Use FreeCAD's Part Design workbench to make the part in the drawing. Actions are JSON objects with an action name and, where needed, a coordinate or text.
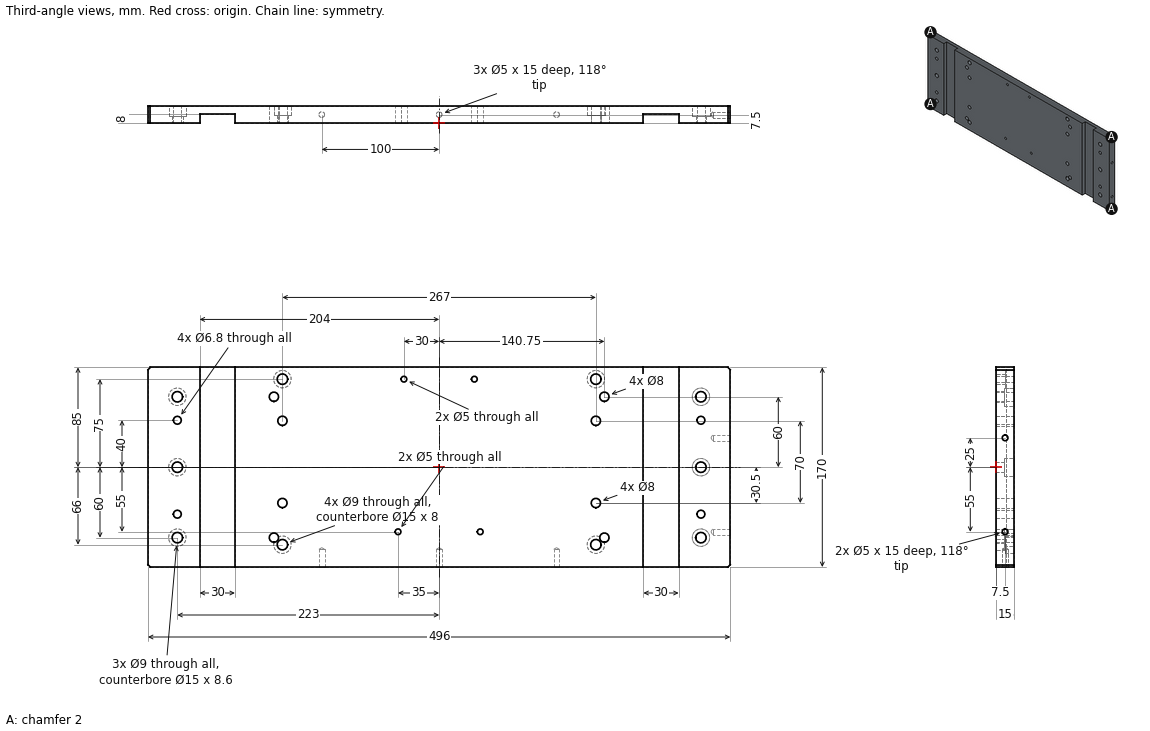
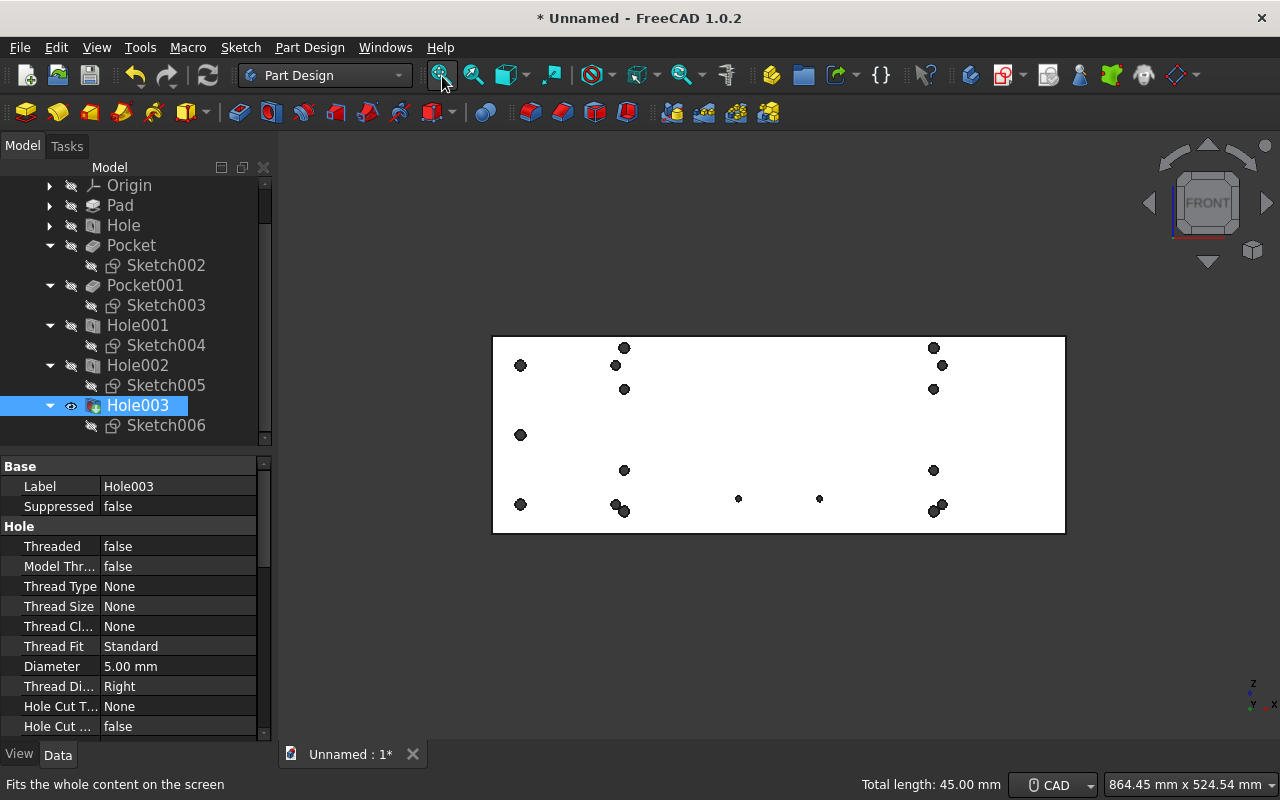
{"action": "key", "text": "3"}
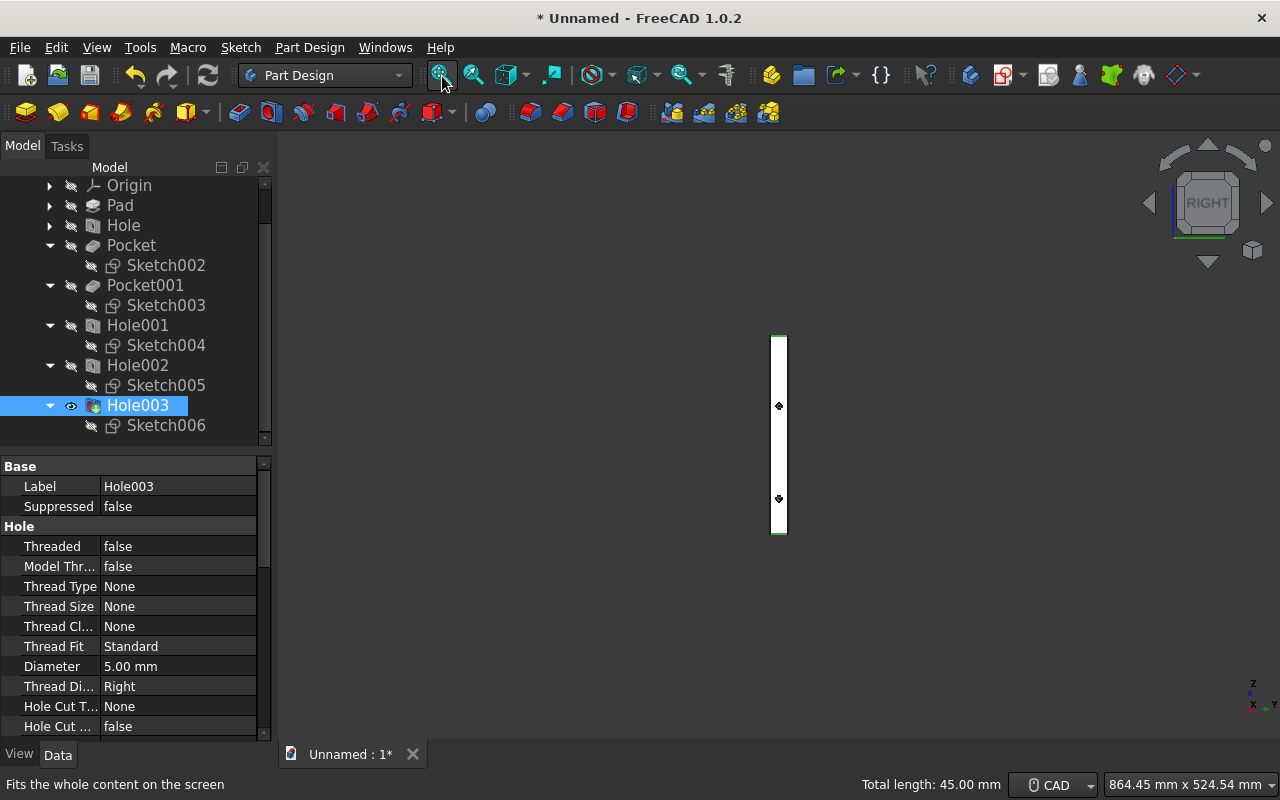
{"action": "left_click", "coordinate": [442, 76]}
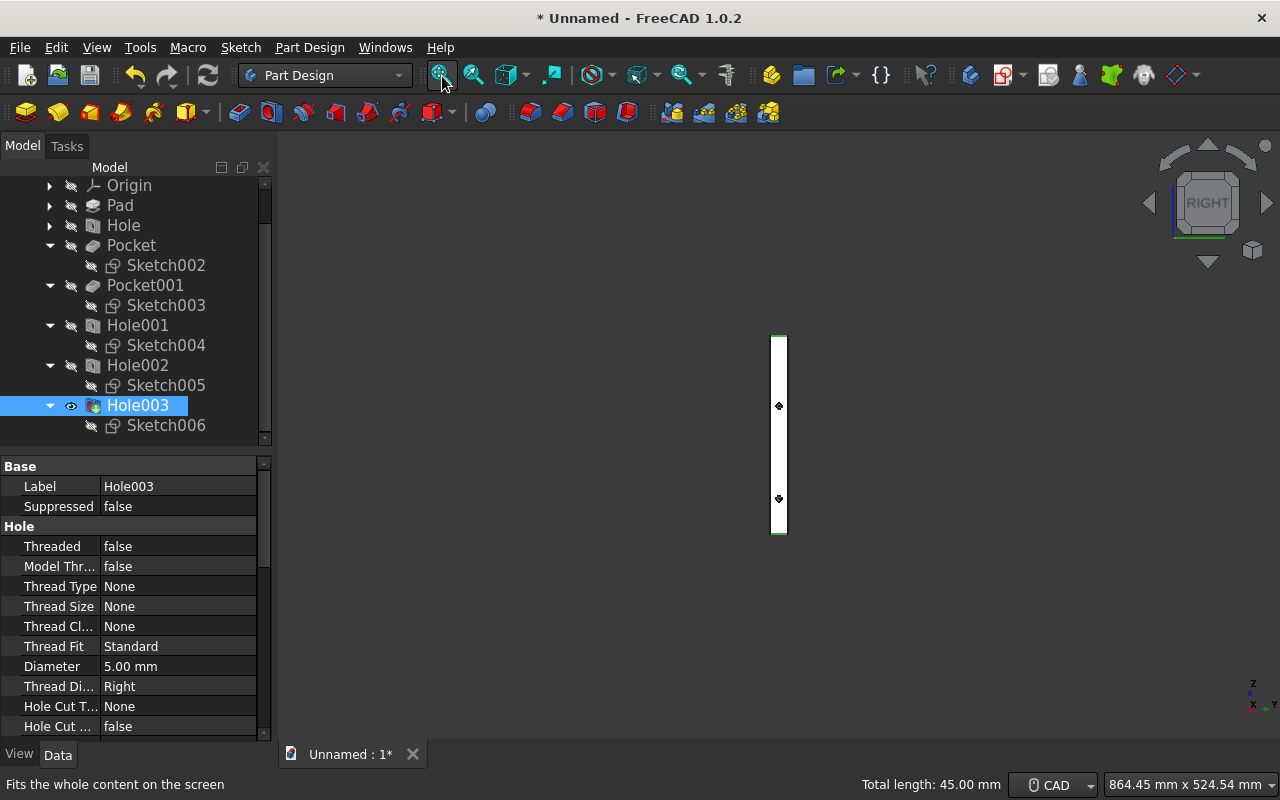
{"action": "scroll", "coordinate": [779, 533], "scroll_direction": "up", "scroll_amount": 5}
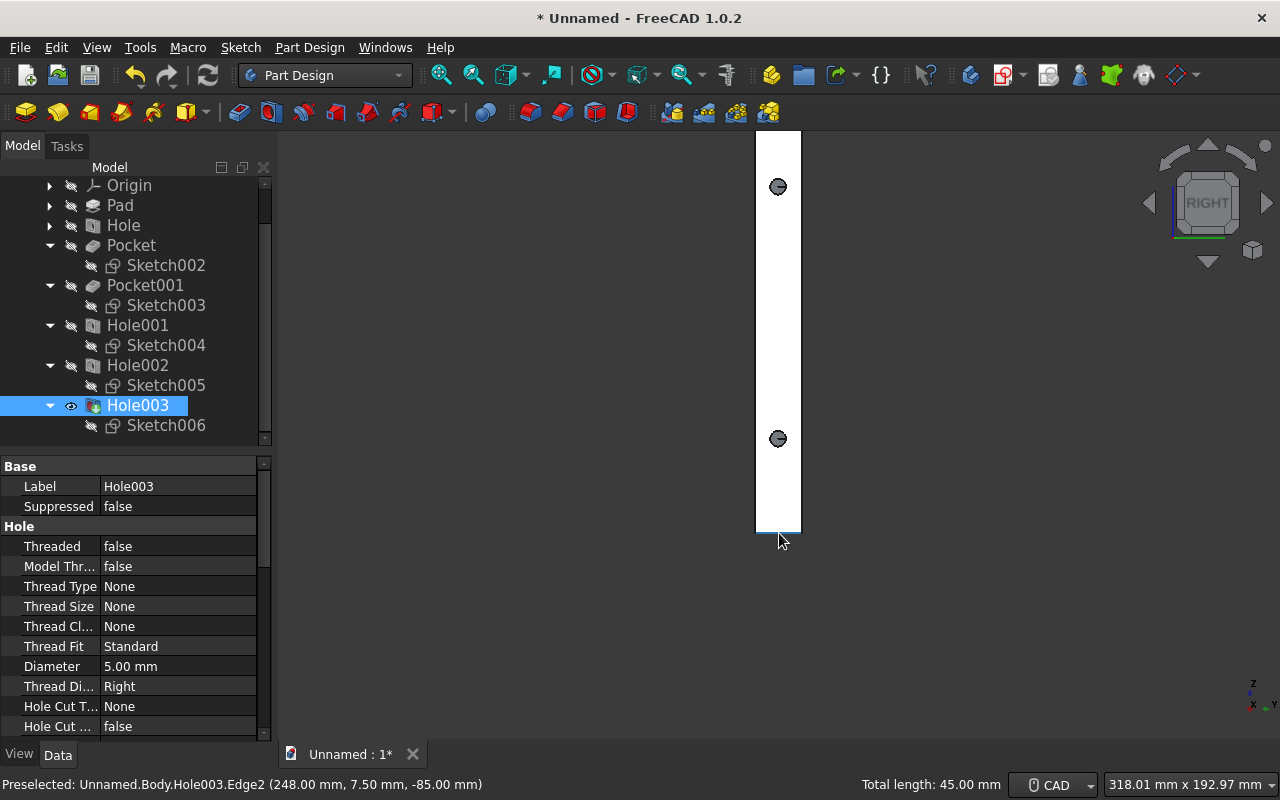
{"action": "left_click", "coordinate": [442, 76]}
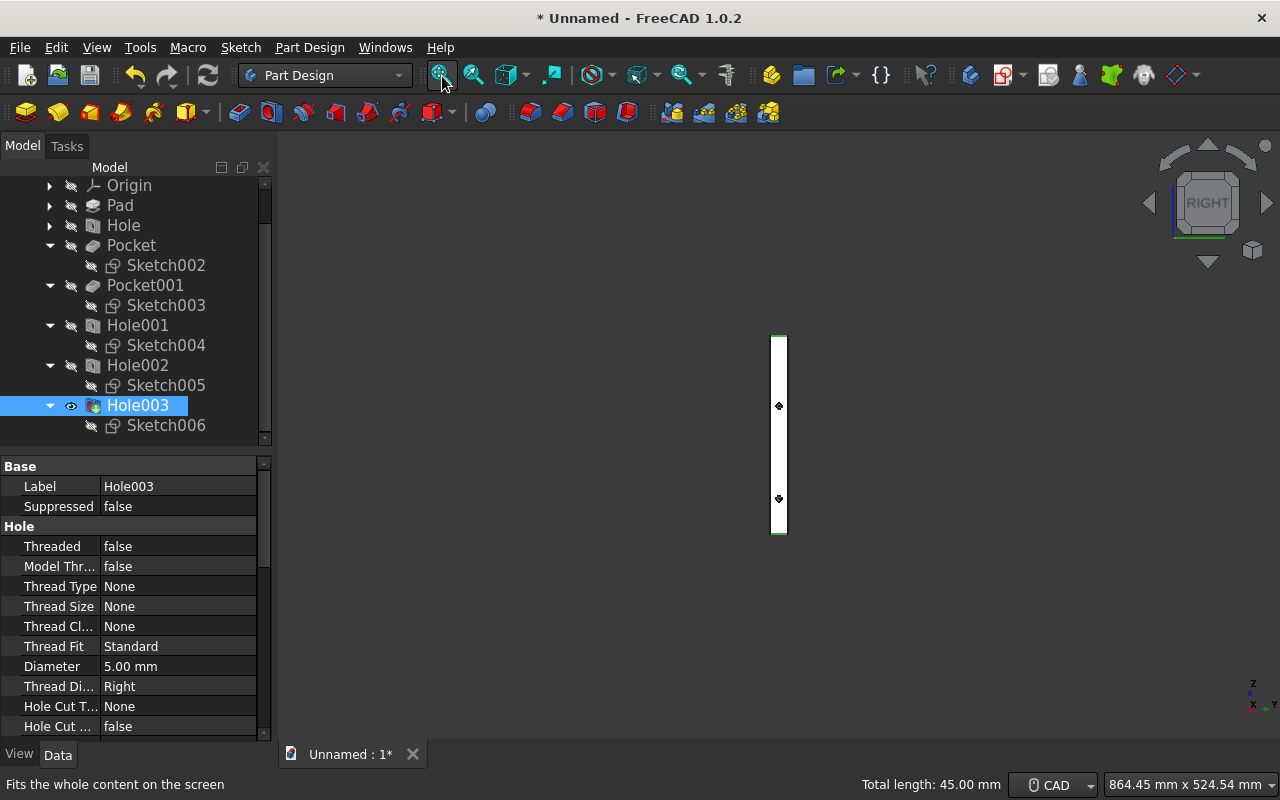
{"action": "key", "text": "5"}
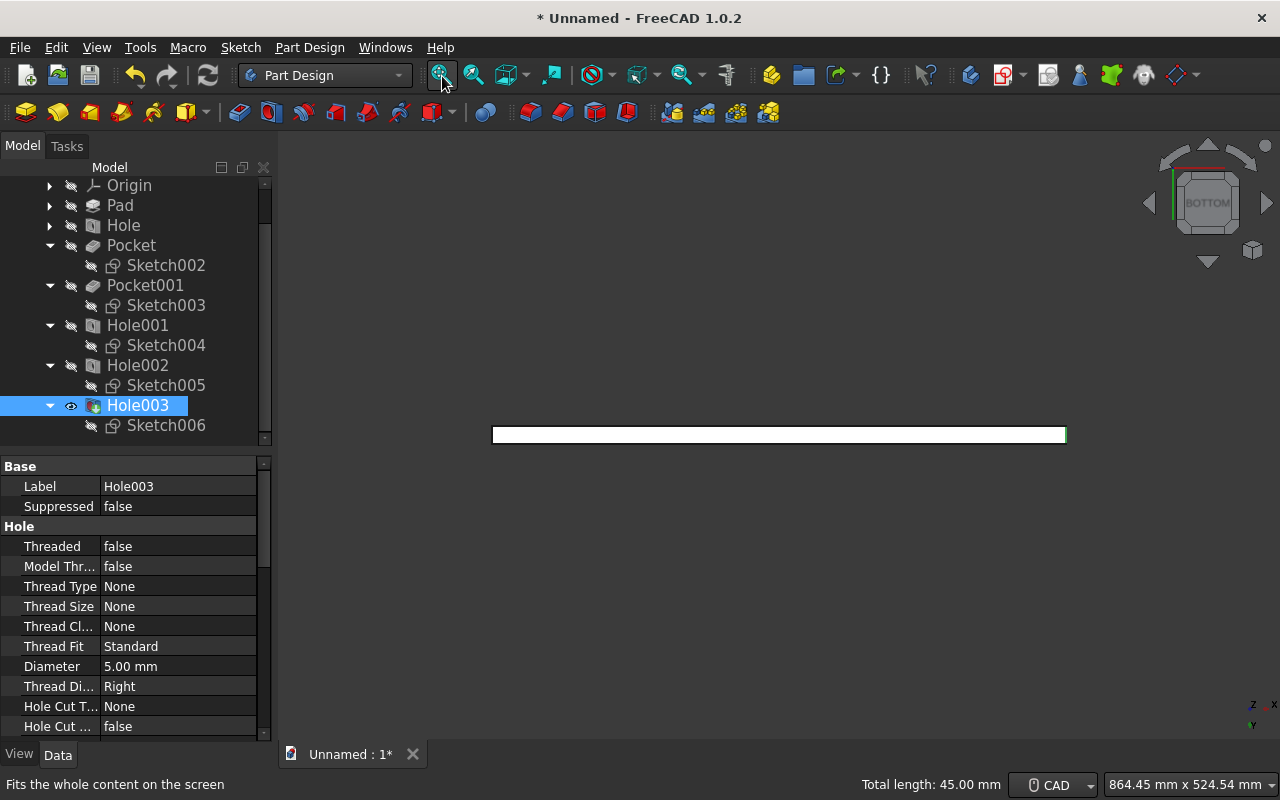
{"action": "left_click", "coordinate": [492, 434], "text": "ctrl"}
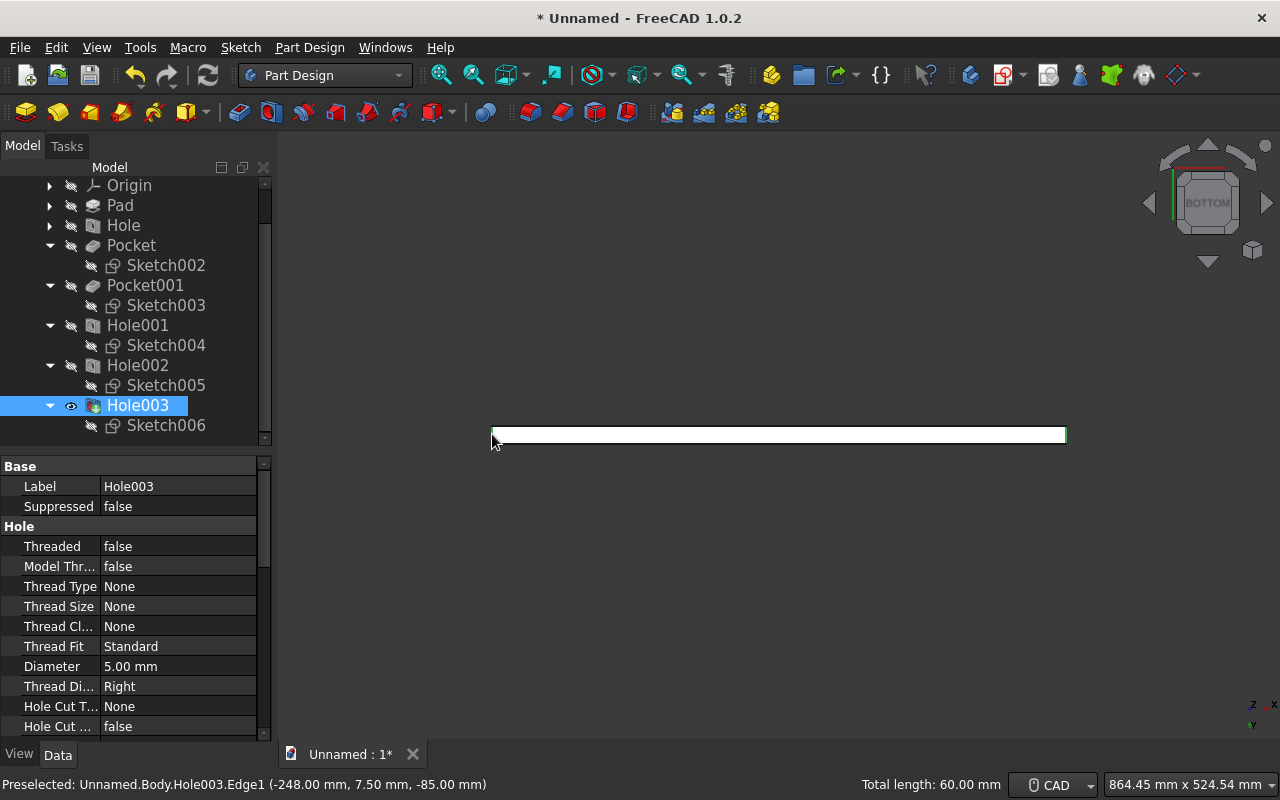
{"action": "left_click", "coordinate": [564, 112]}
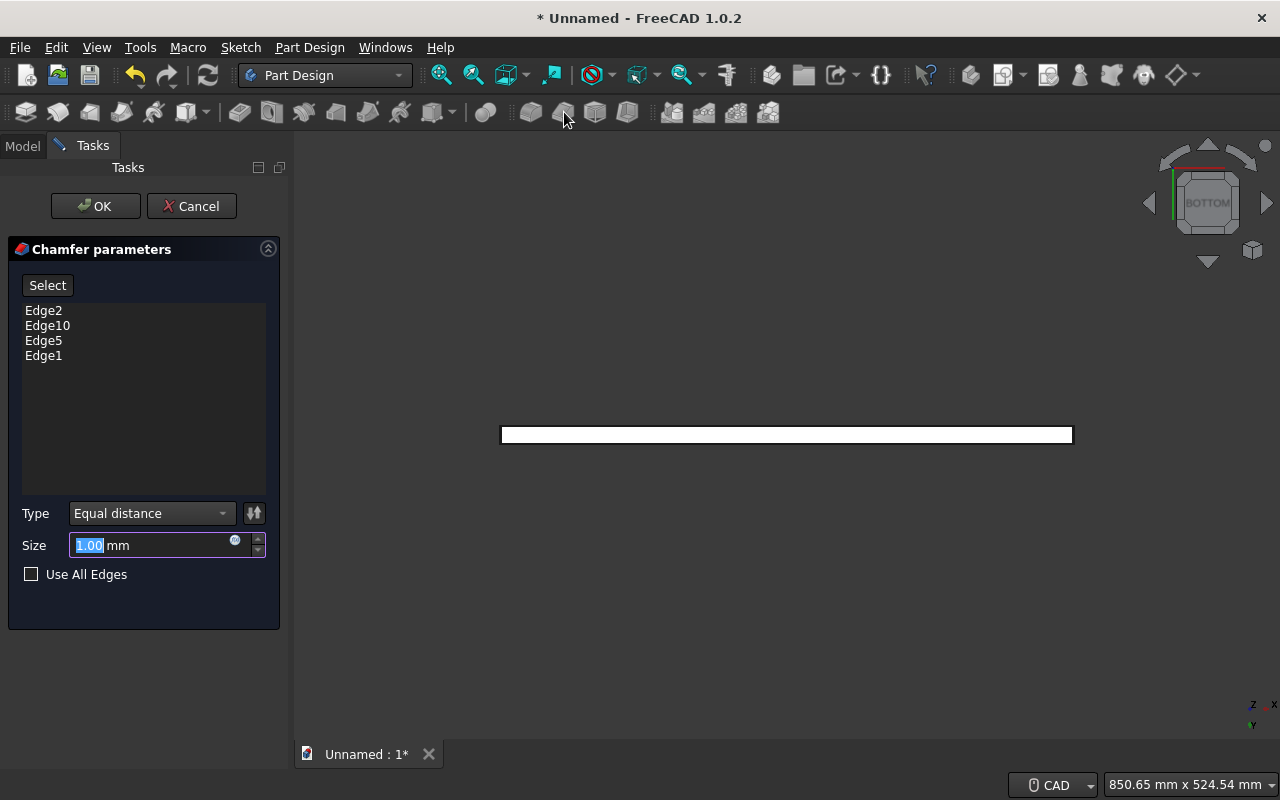
{"action": "type", "text": "2"}
{"action": "key", "text": "Tab"}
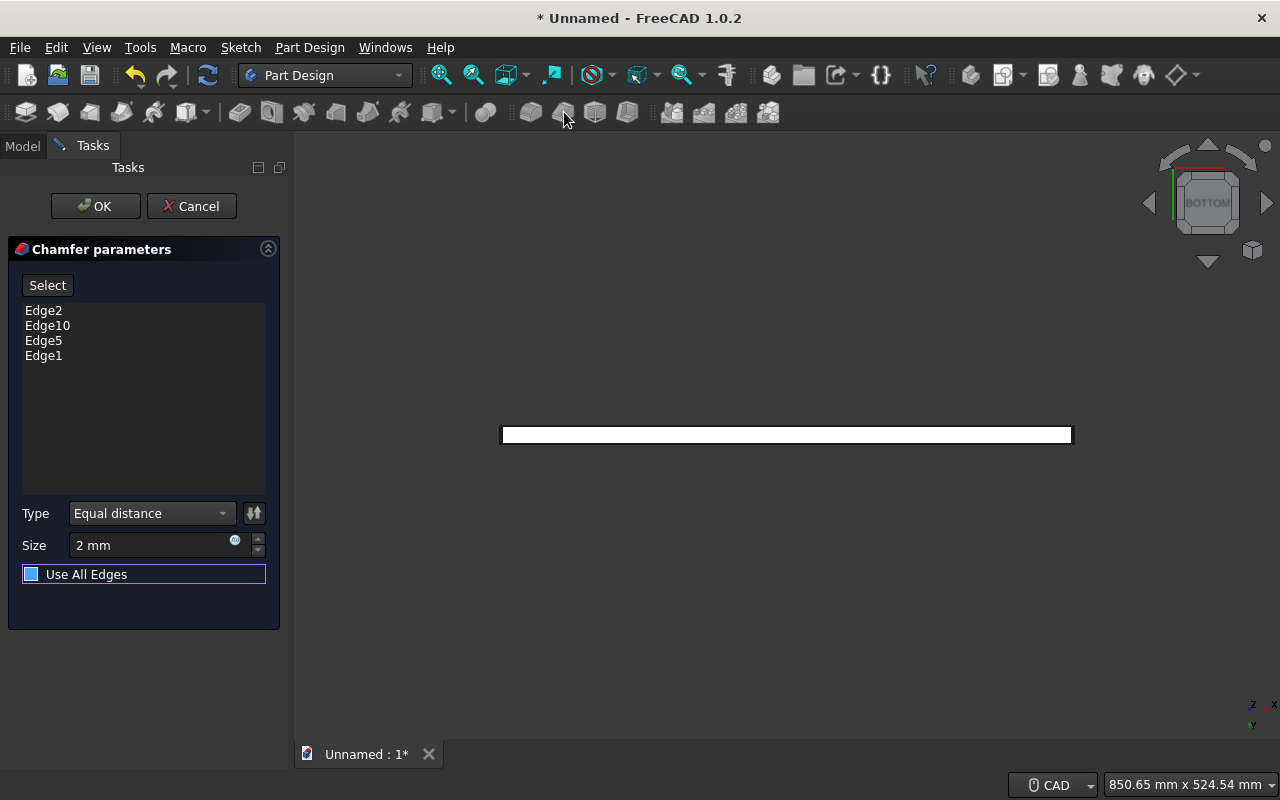
{"action": "left_click", "coordinate": [96, 206]}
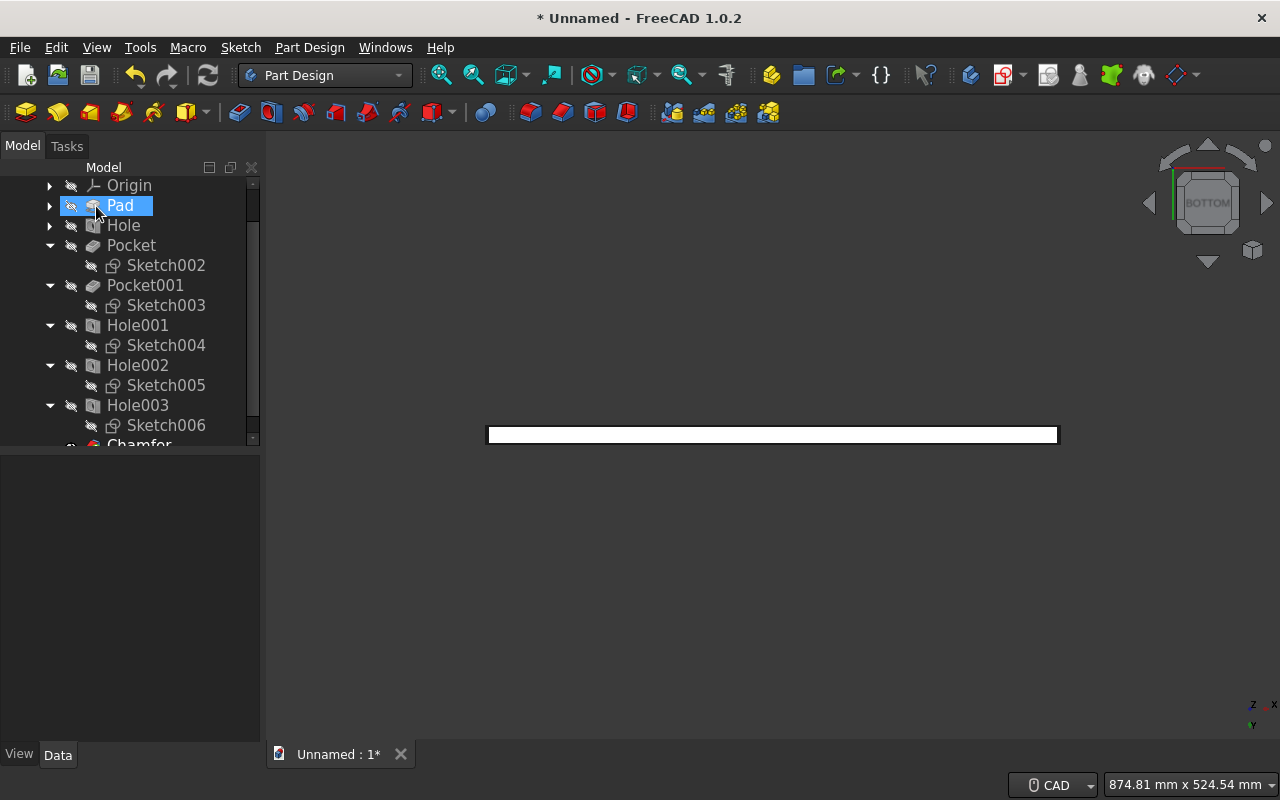
{"action": "key", "text": "0"}